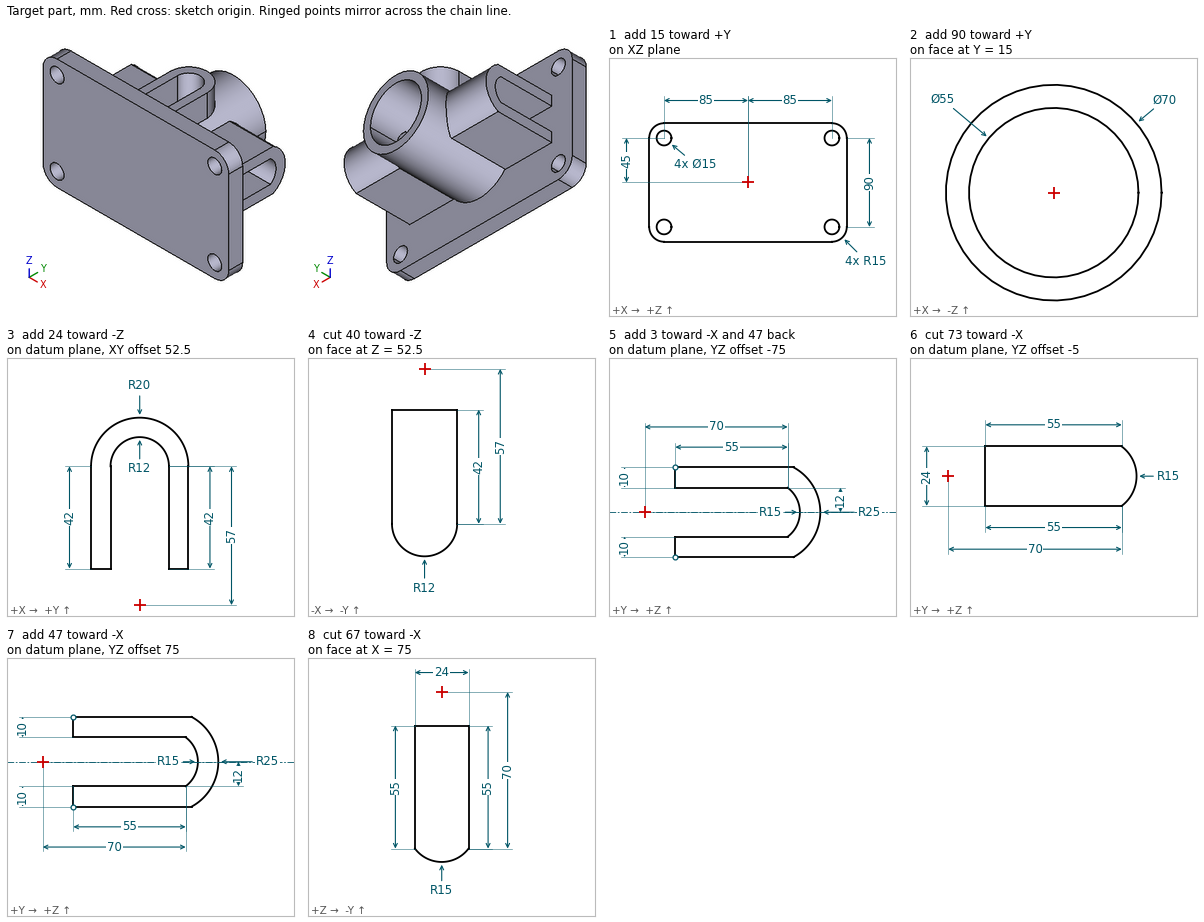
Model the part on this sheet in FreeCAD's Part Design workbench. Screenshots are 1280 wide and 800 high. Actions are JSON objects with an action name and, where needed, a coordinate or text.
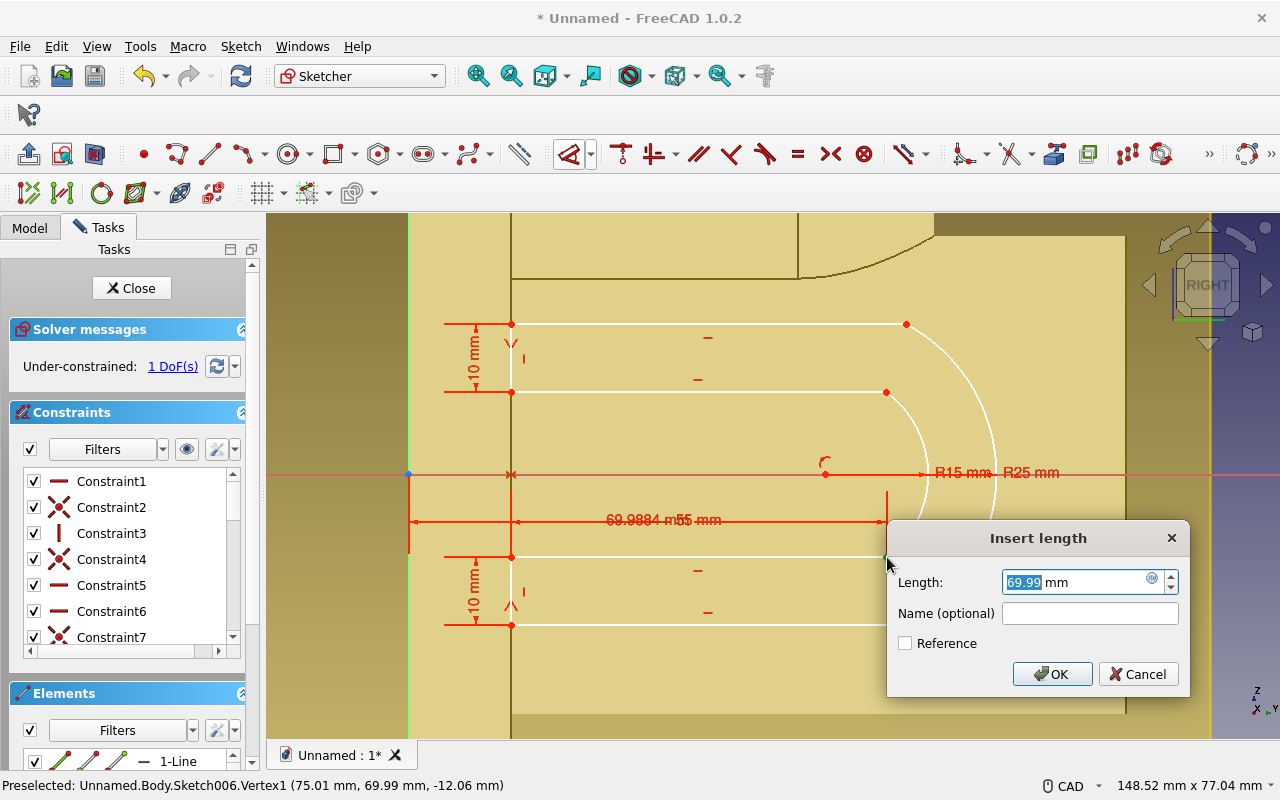
{"action": "type", "text": "70"}
{"action": "key", "text": "Return"}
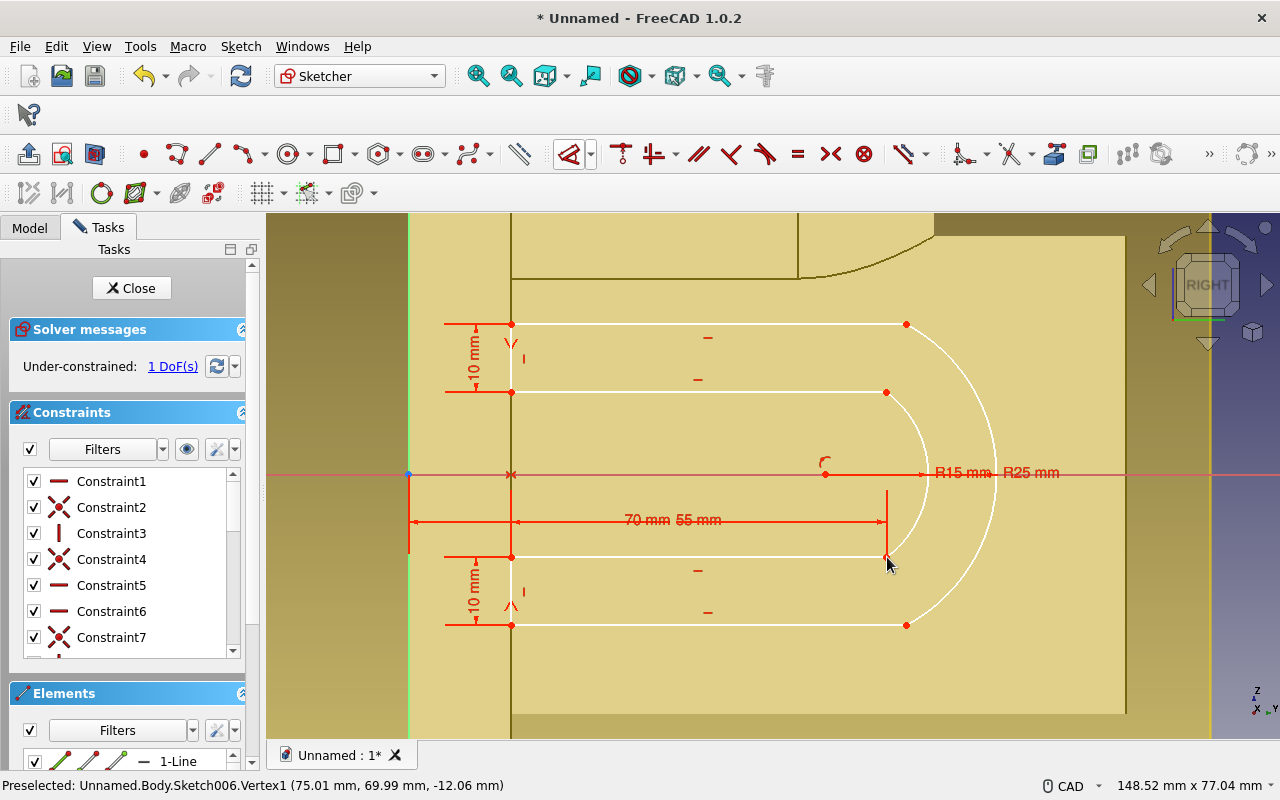
{"action": "left_click", "coordinate": [887, 557]}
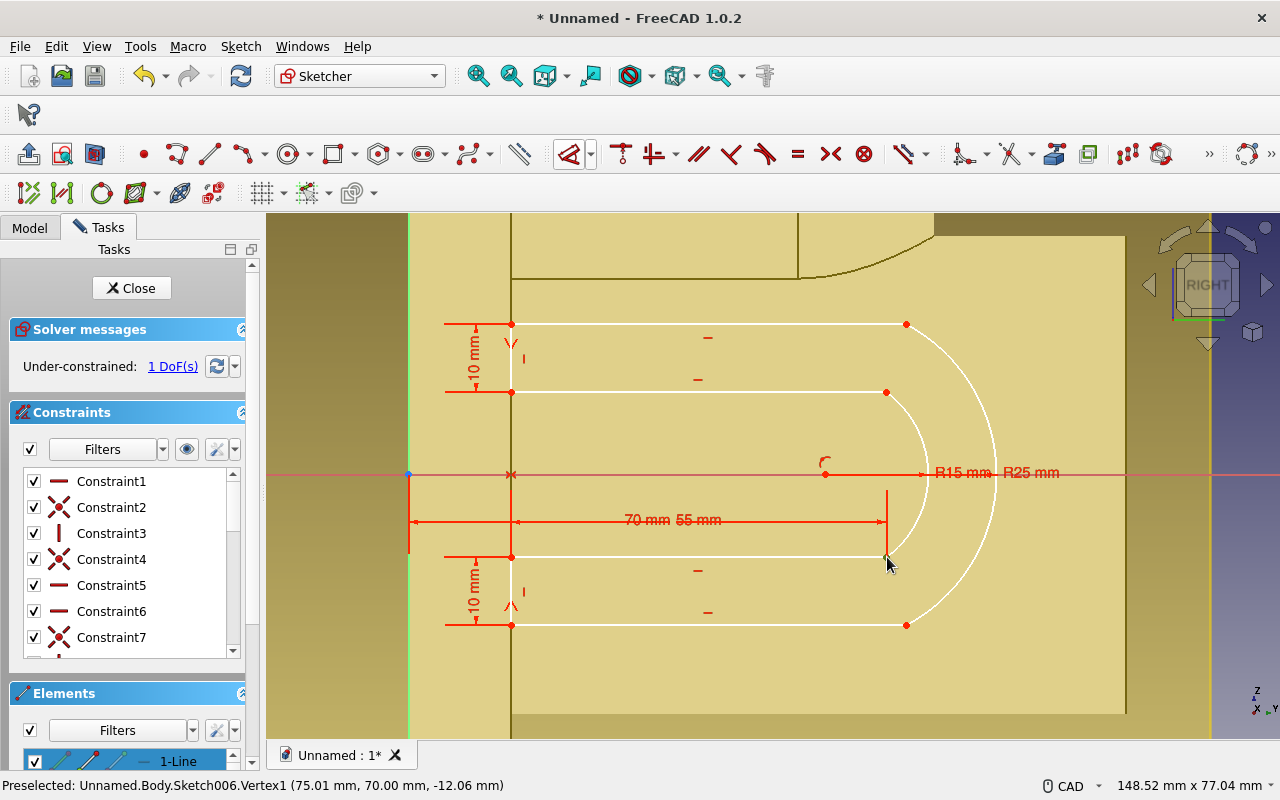
{"action": "key", "text": "i"}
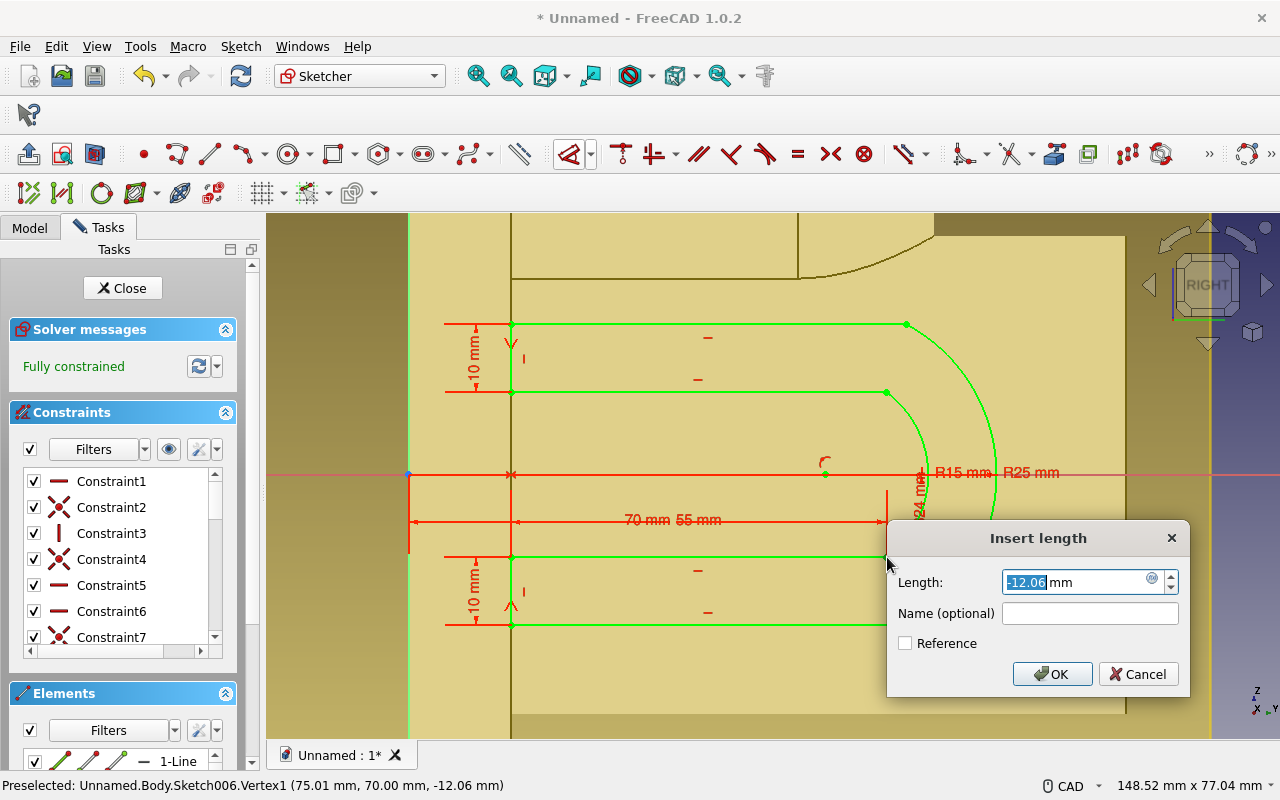
{"action": "type", "text": "-12"}
{"action": "key", "text": "Return"}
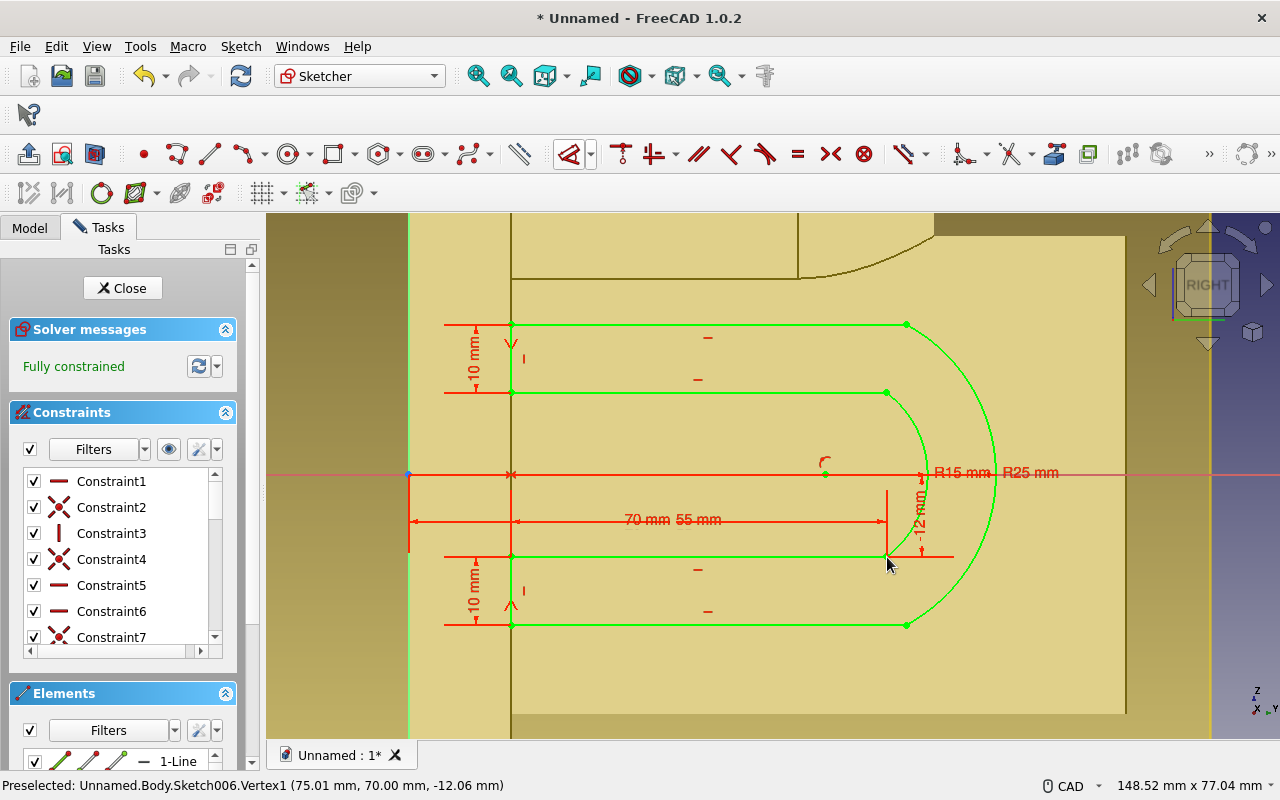
{"action": "left_click", "coordinate": [123, 288]}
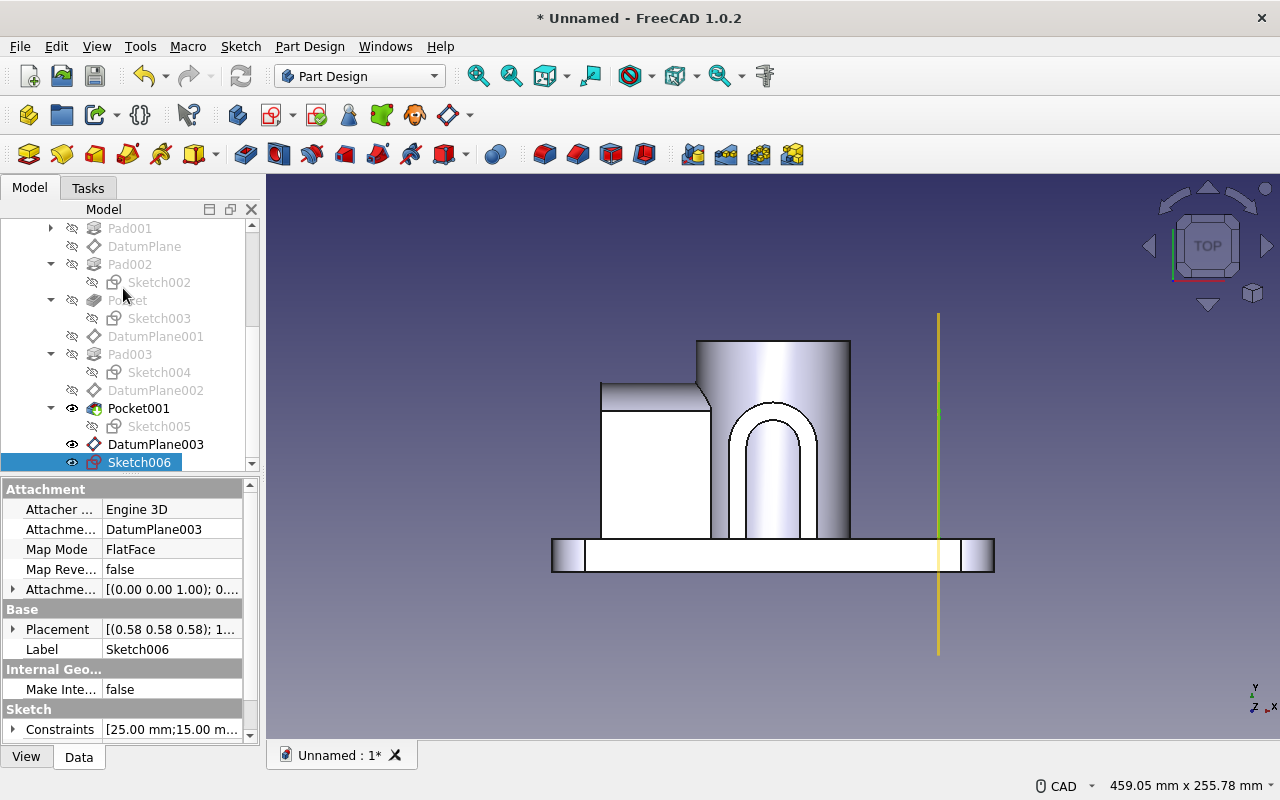
{"action": "left_click", "coordinate": [29, 154]}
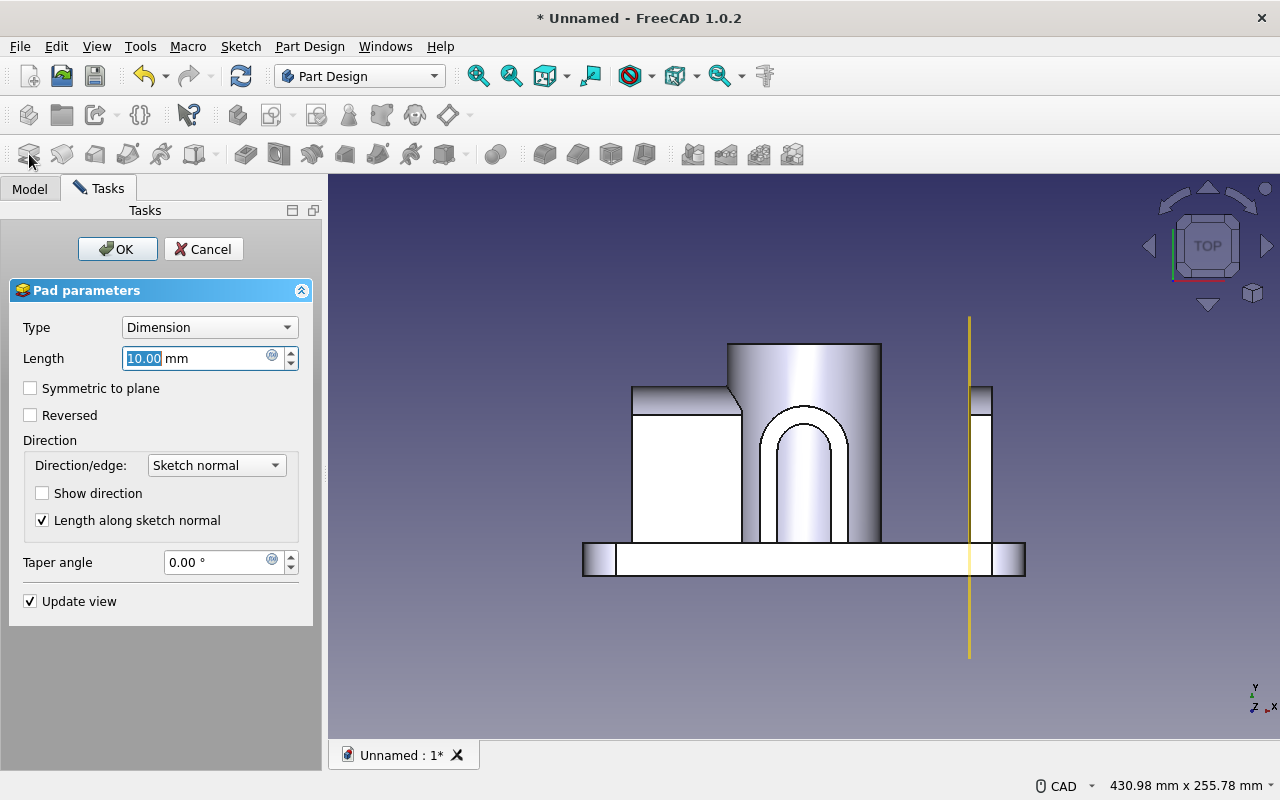
{"action": "type", "text": "47"}
{"action": "key", "text": "Tab"}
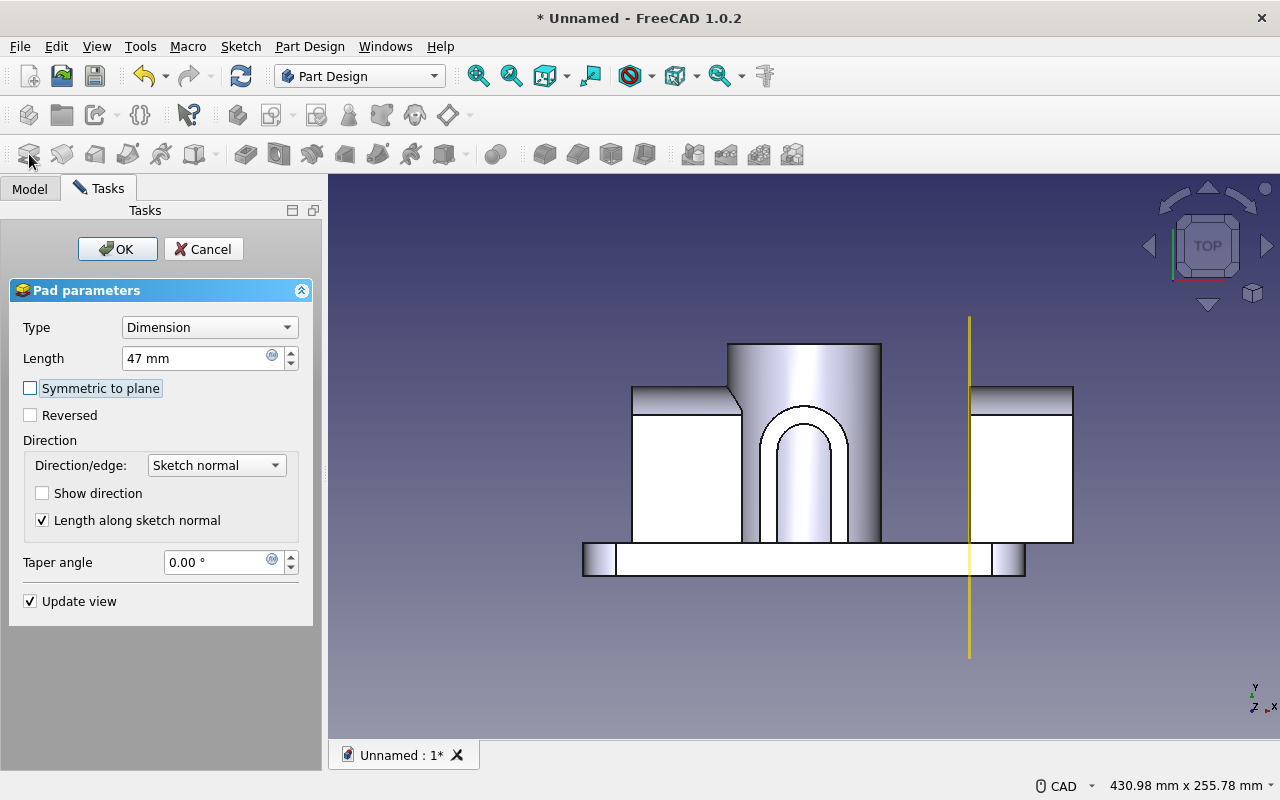
{"action": "left_click", "coordinate": [31, 415]}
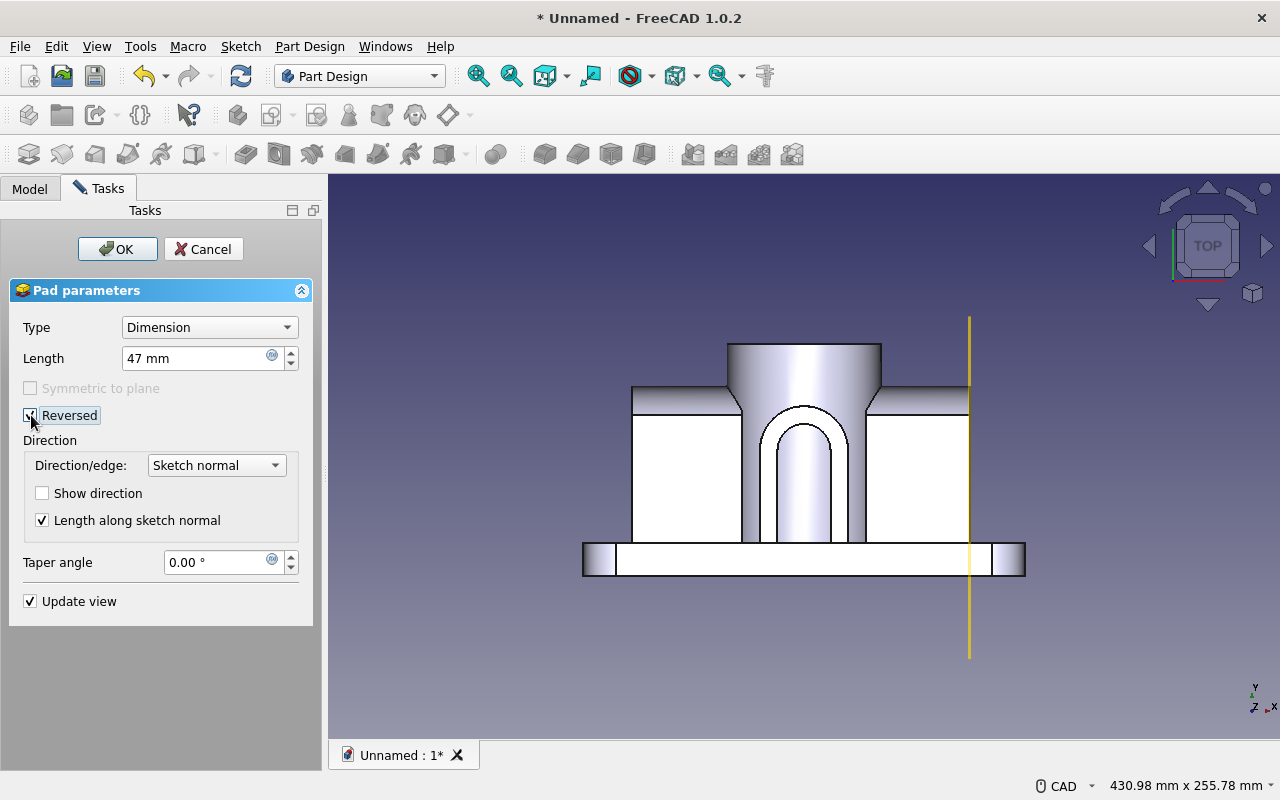
{"action": "left_click", "coordinate": [118, 249]}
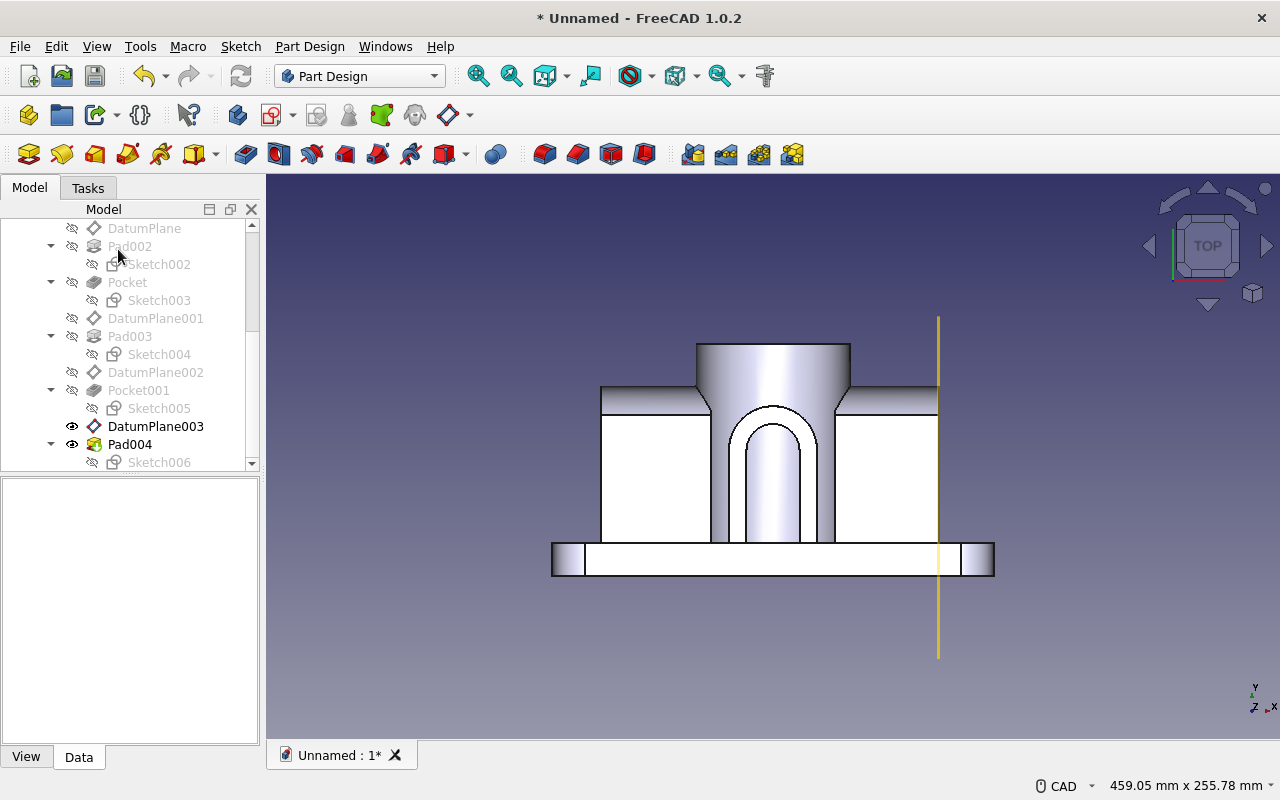
{"action": "left_click", "coordinate": [117, 426]}
{"action": "key", "text": "space"}